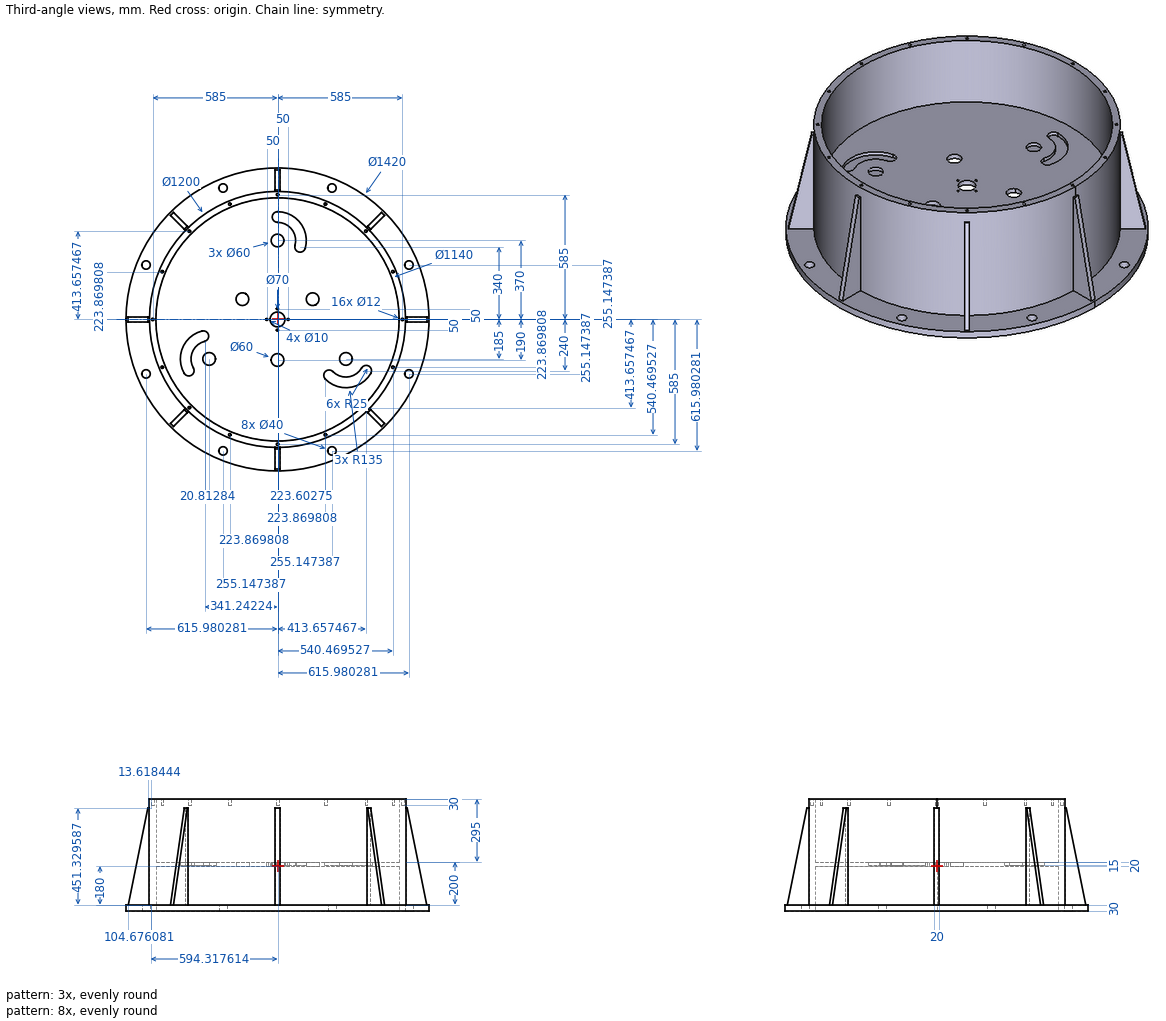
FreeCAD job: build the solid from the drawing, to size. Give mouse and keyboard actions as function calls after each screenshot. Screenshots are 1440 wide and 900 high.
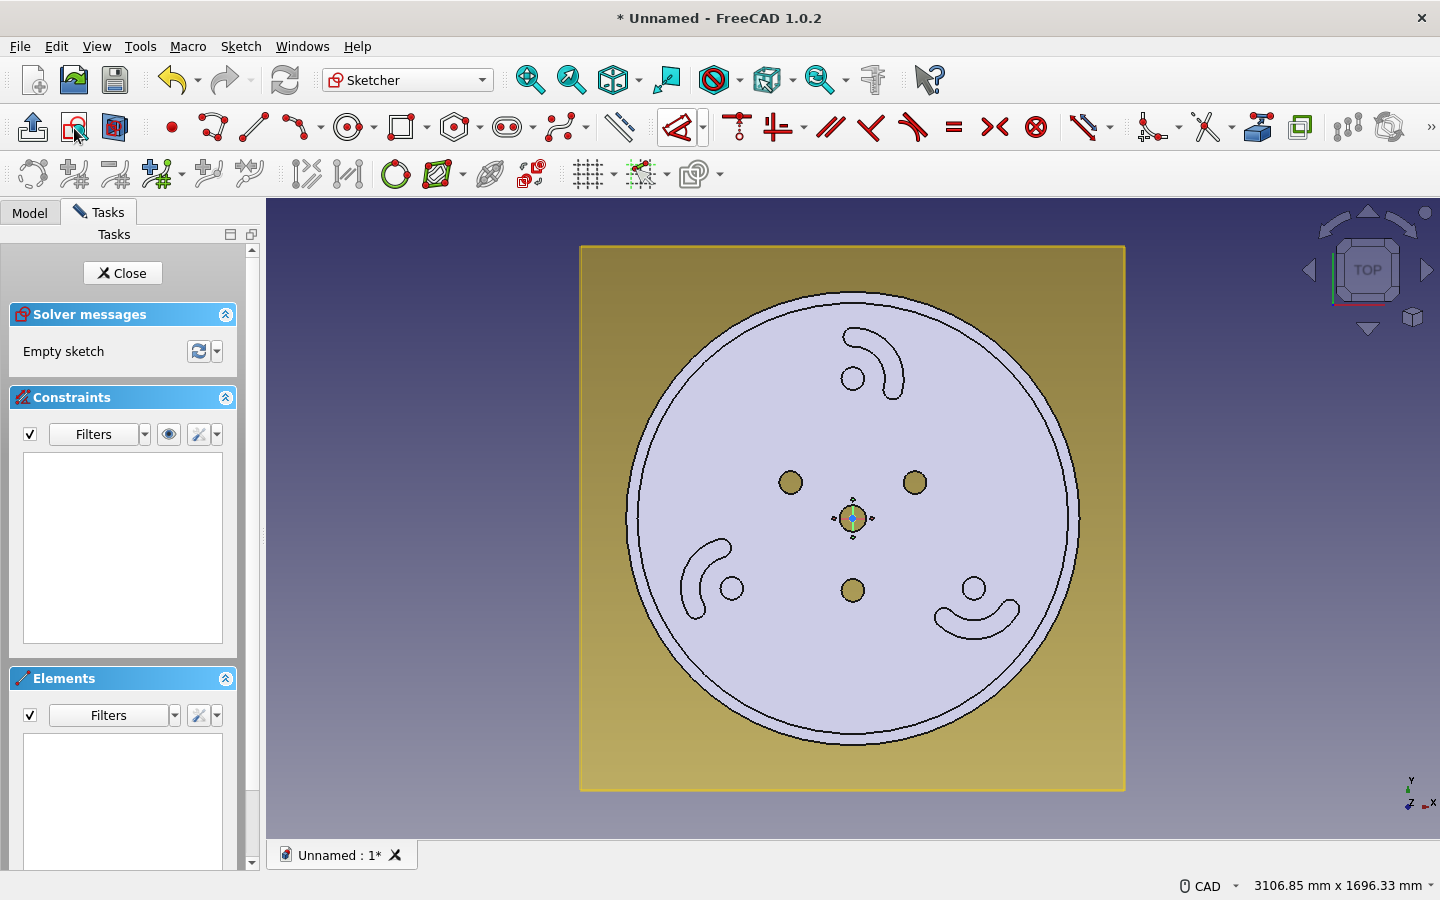
click(115, 128)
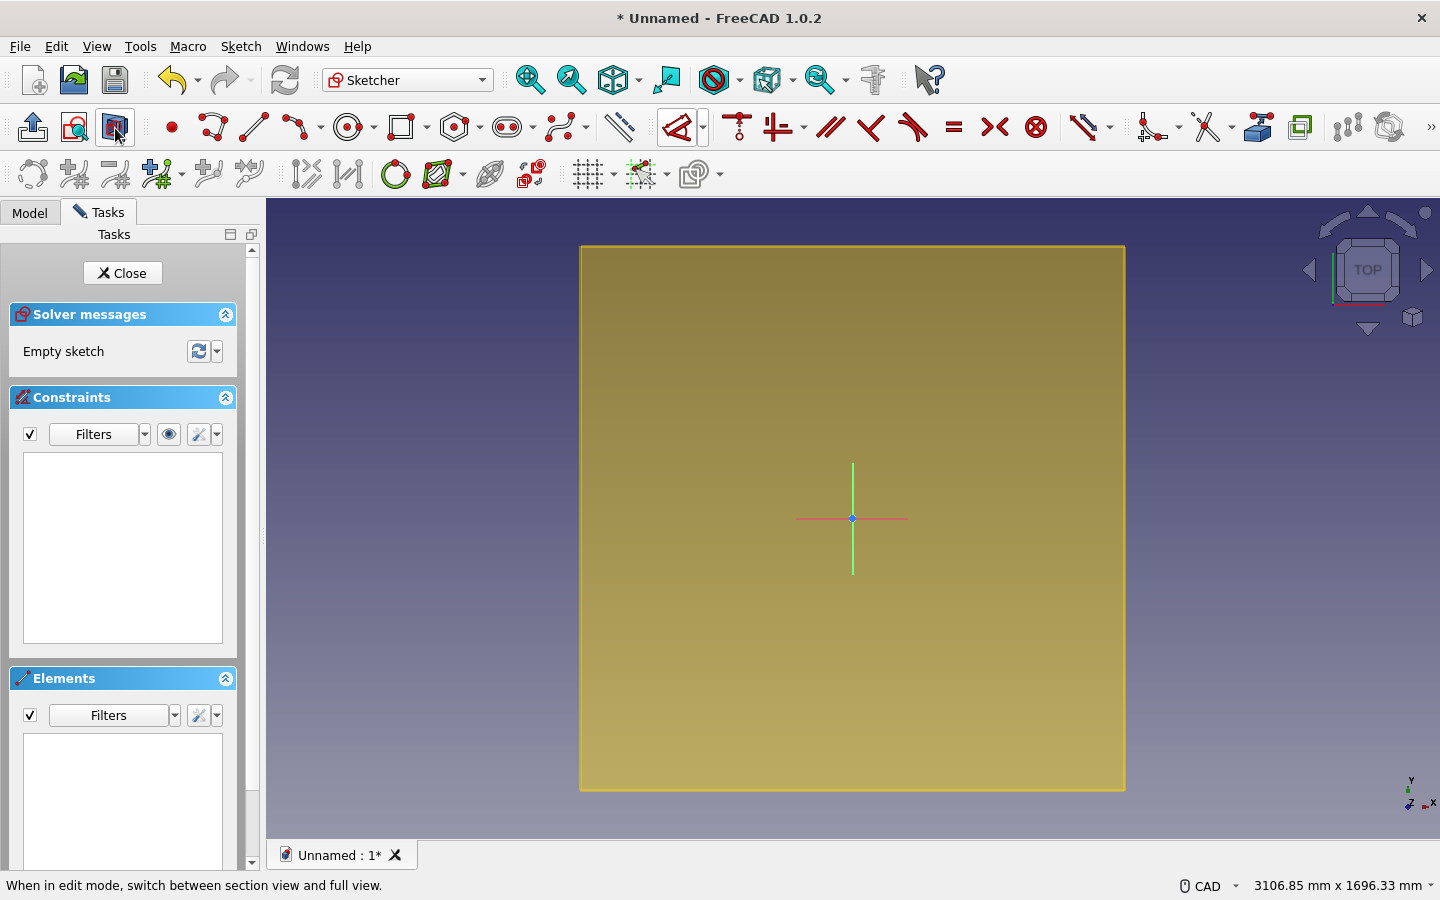
scroll(476, 519, down, 1)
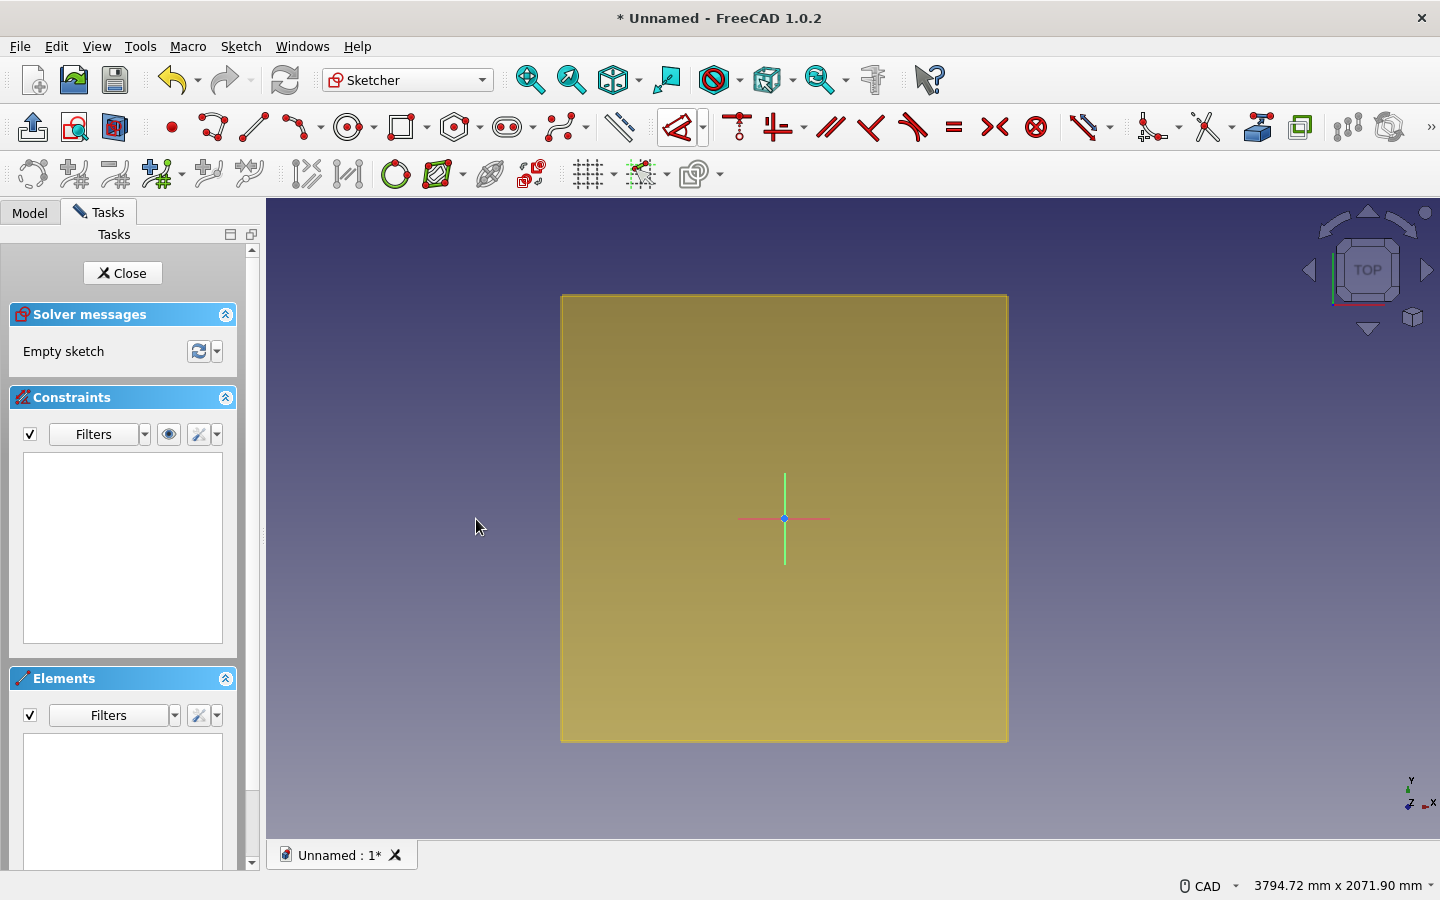
click(348, 128)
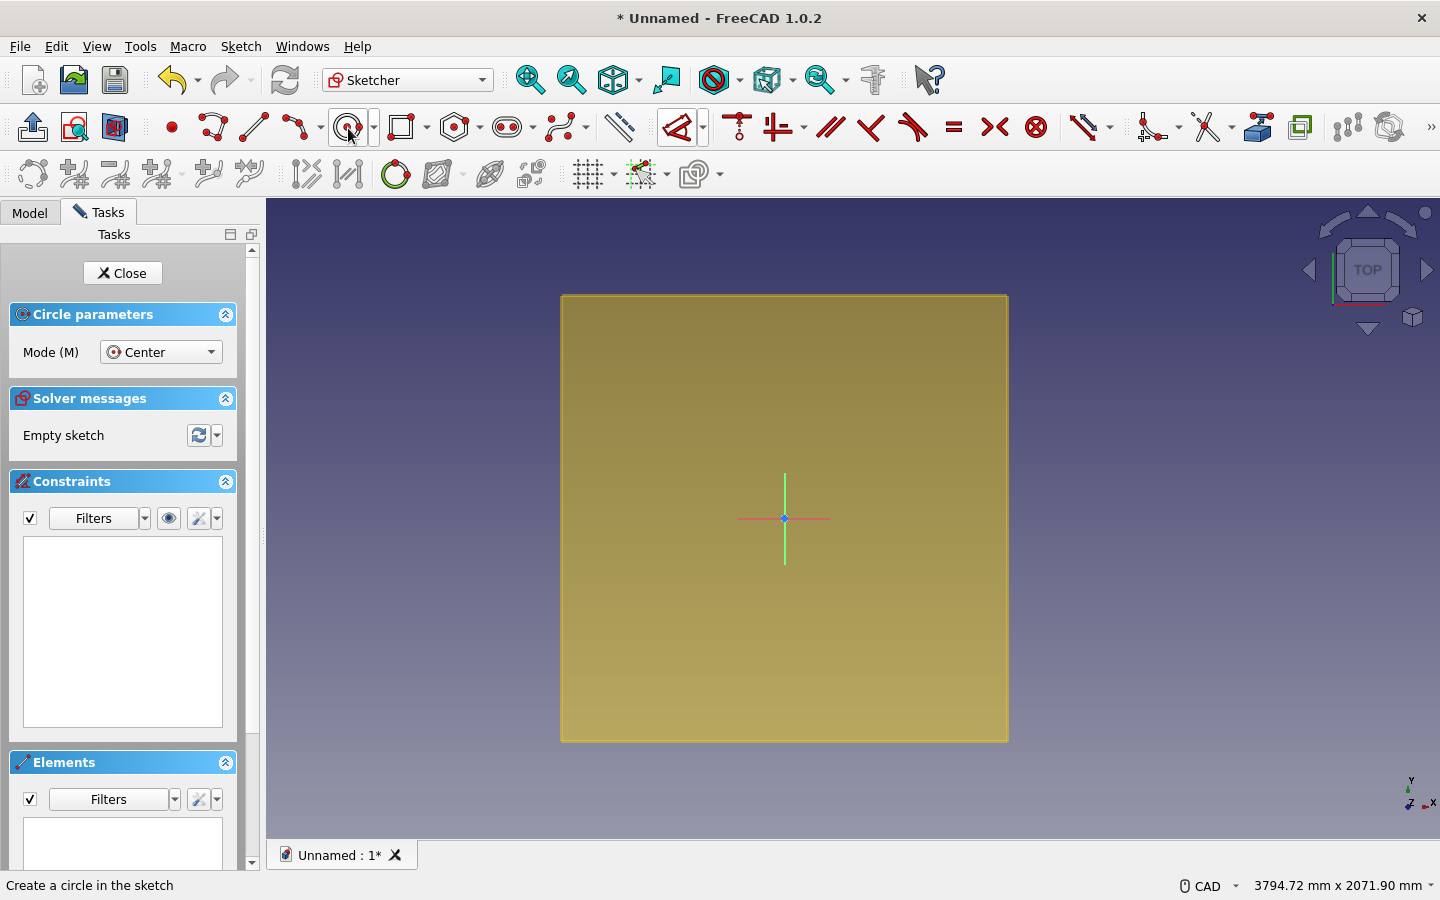
click(785, 519)
move(940, 363)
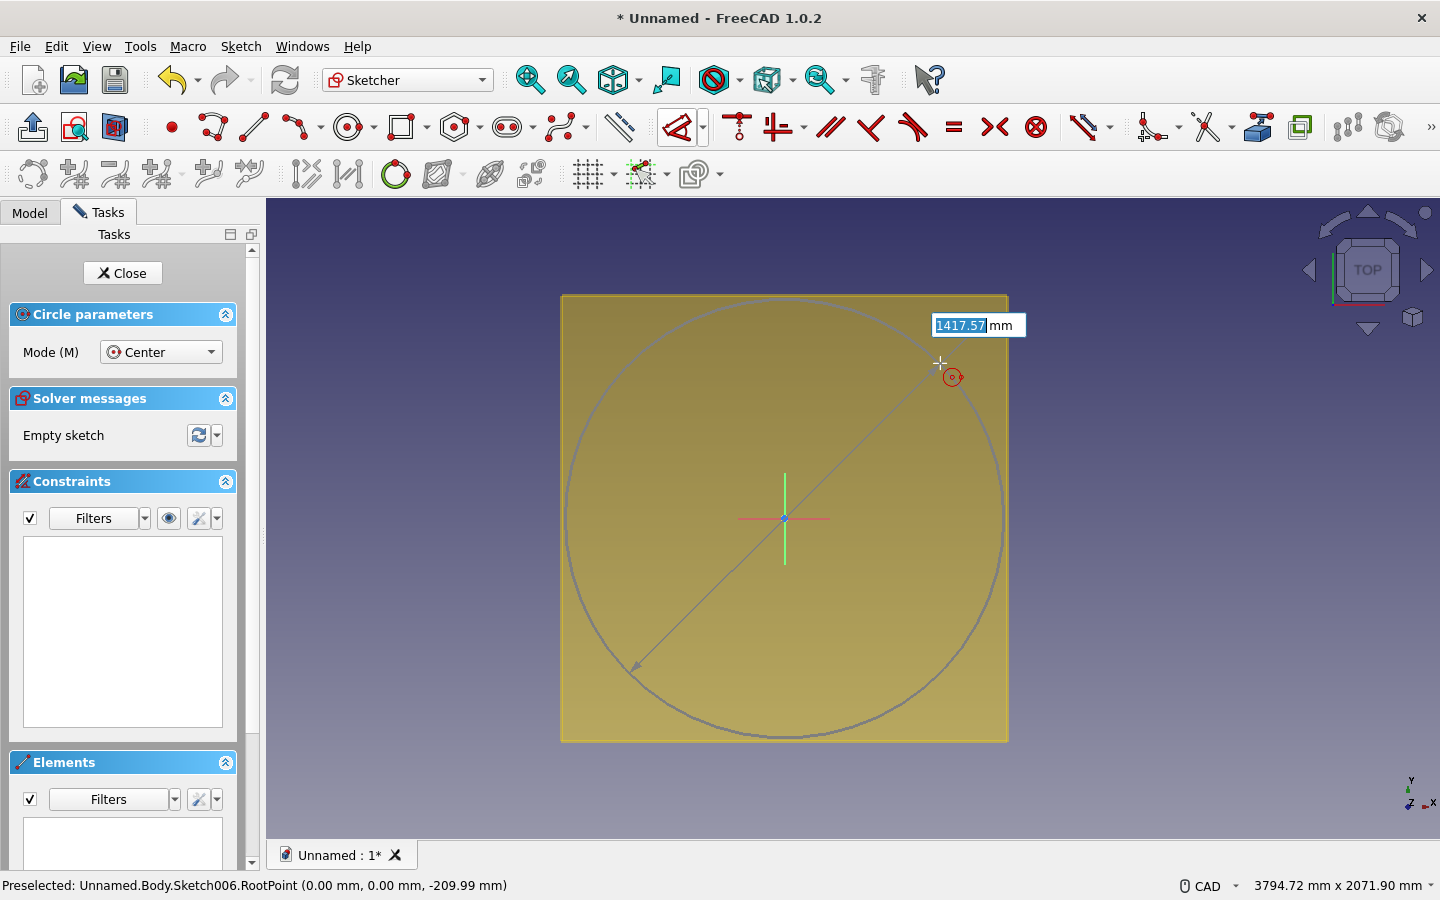
text(1420)
key(Return)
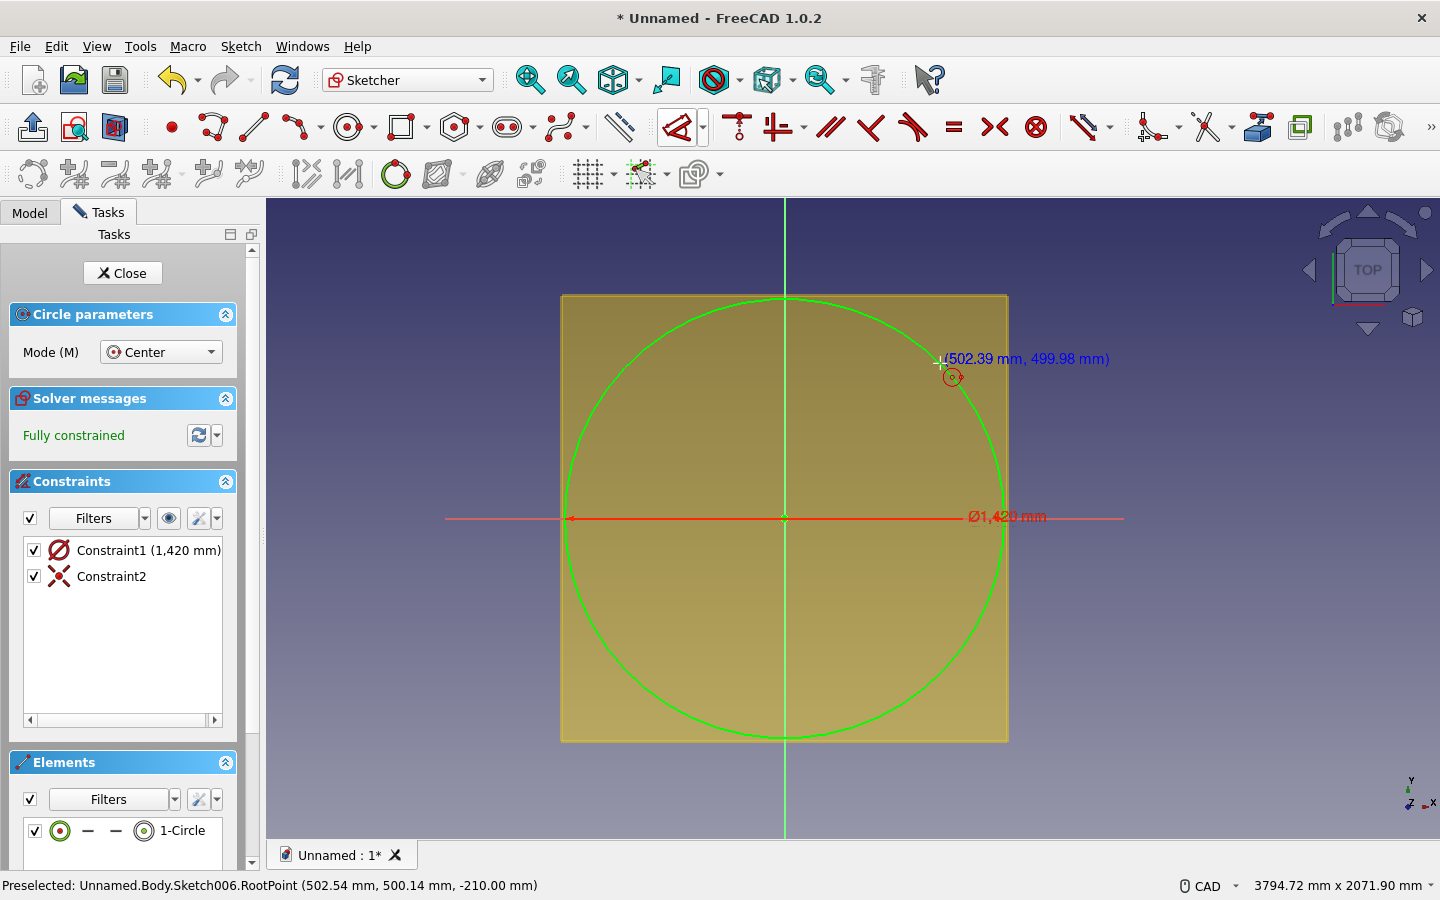
scroll(864, 709, up, 7)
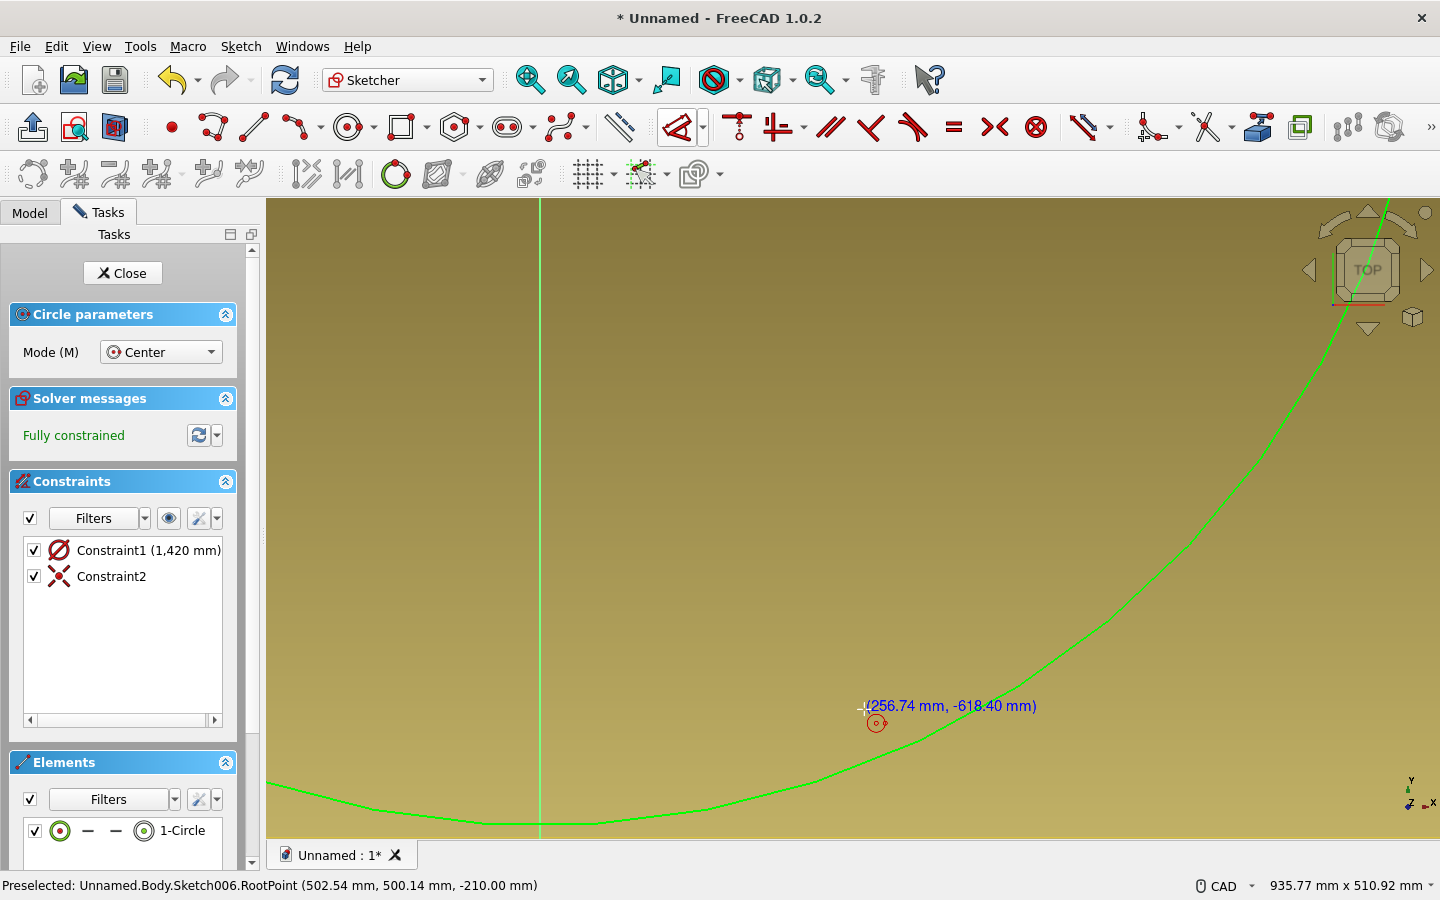
scroll(864, 710, down, 7)